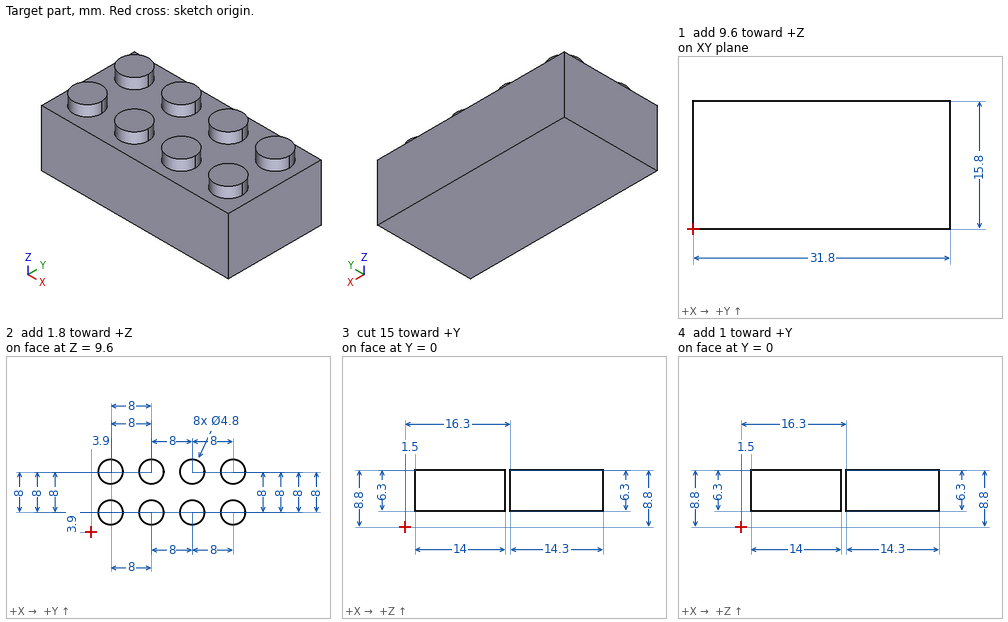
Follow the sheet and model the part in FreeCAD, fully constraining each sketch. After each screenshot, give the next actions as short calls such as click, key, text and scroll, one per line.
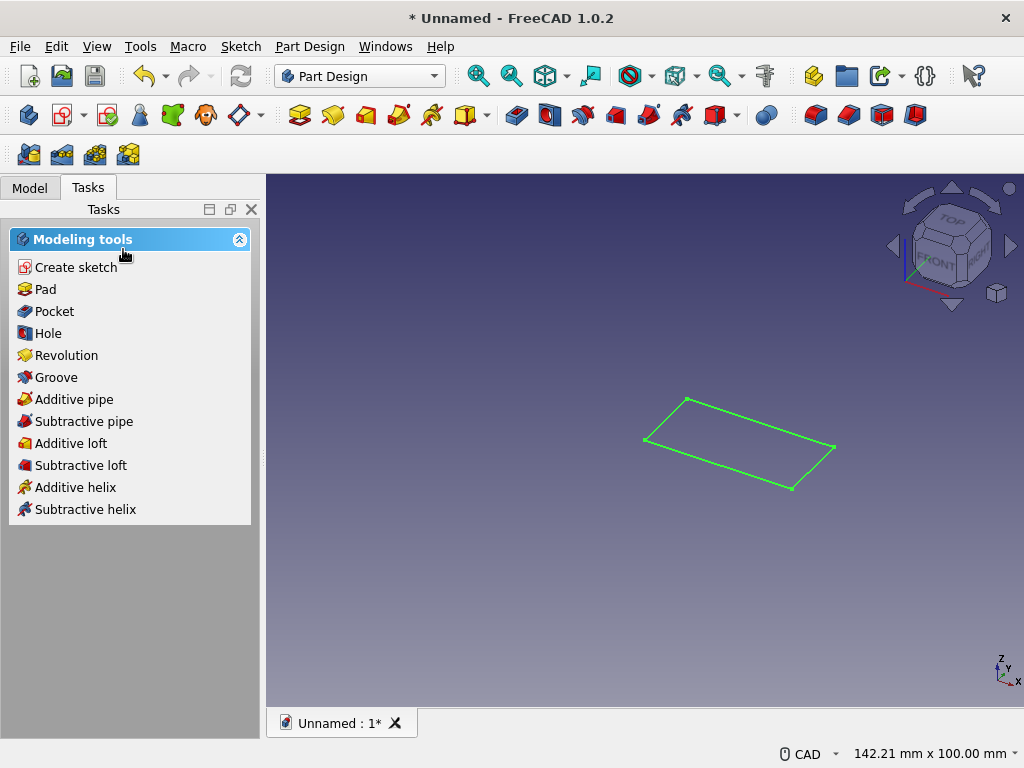
click(300, 116)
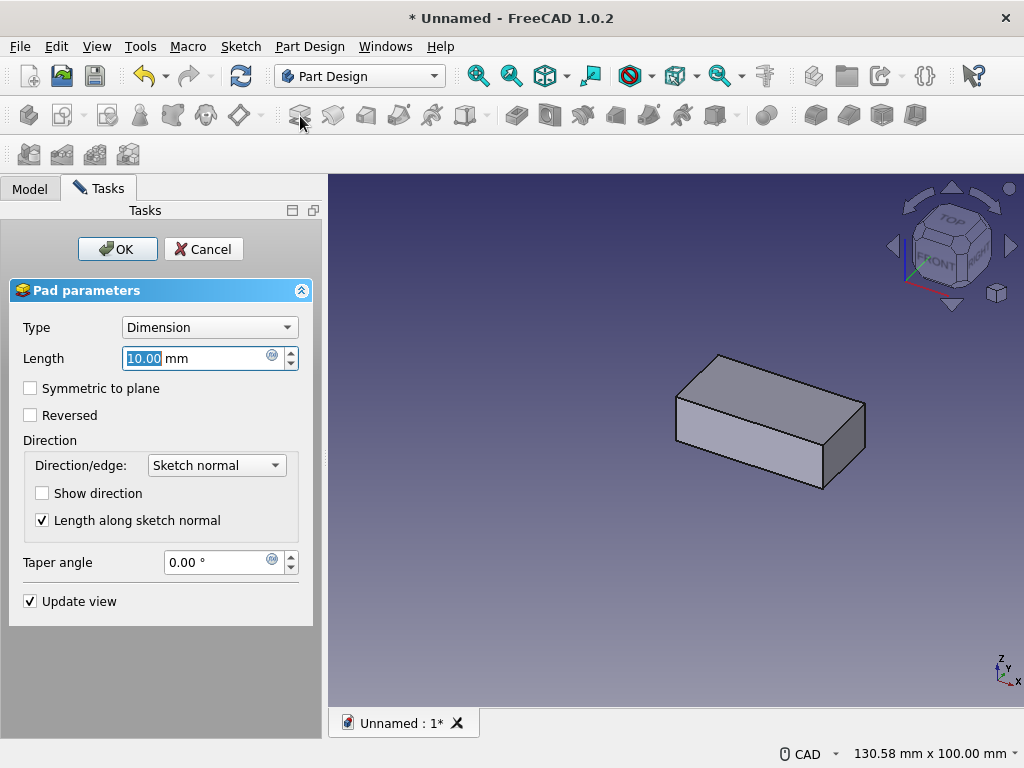
text(9.6)
key(Tab)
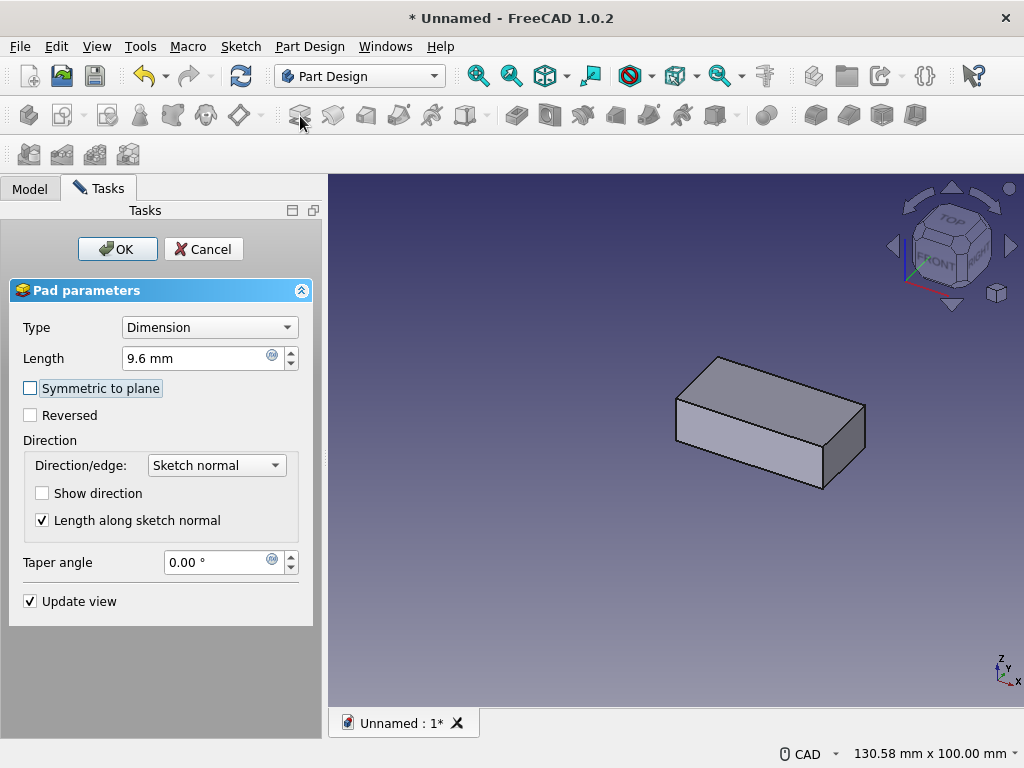
click(118, 249)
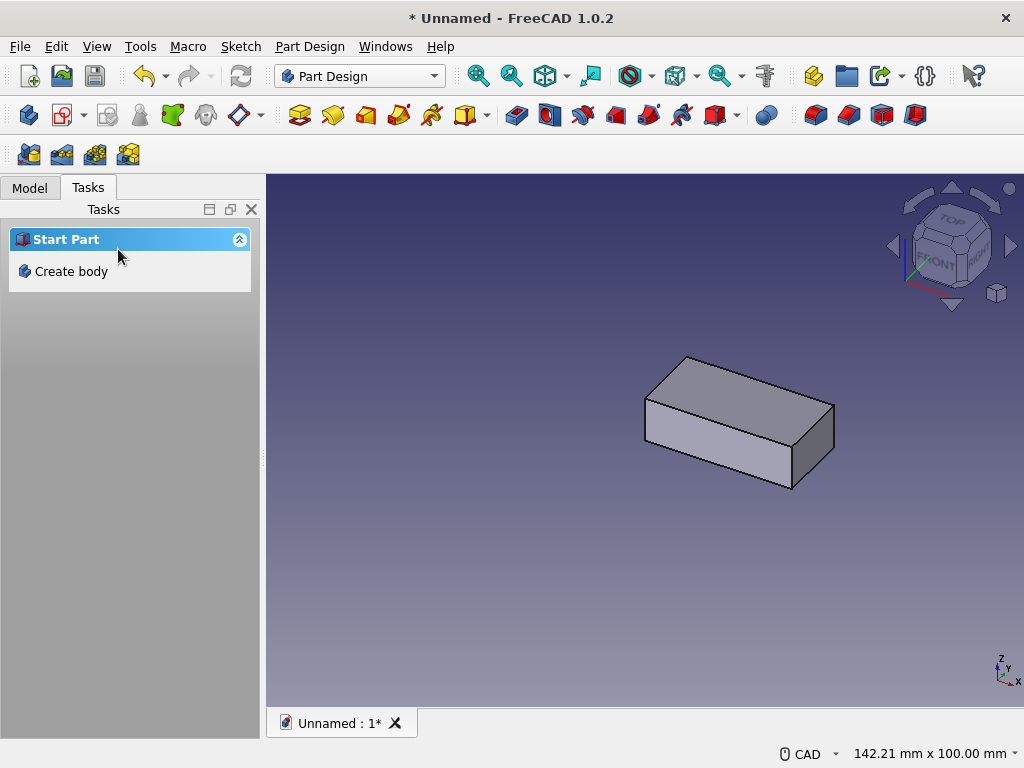
key(v)
key(f)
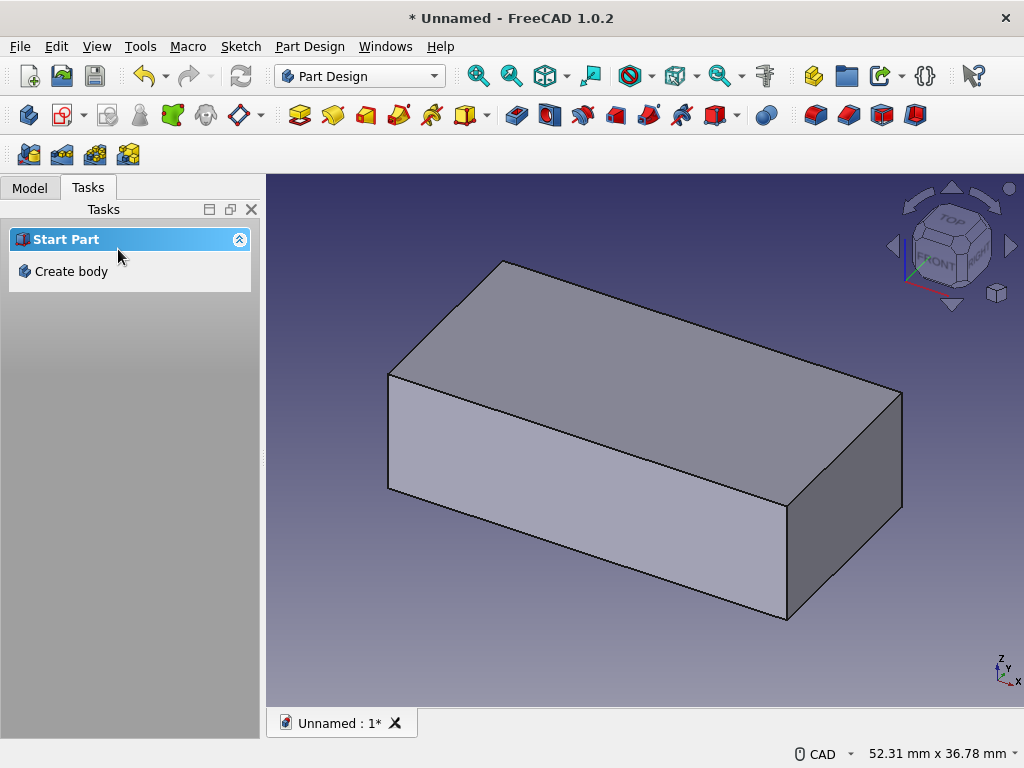
click(702, 401)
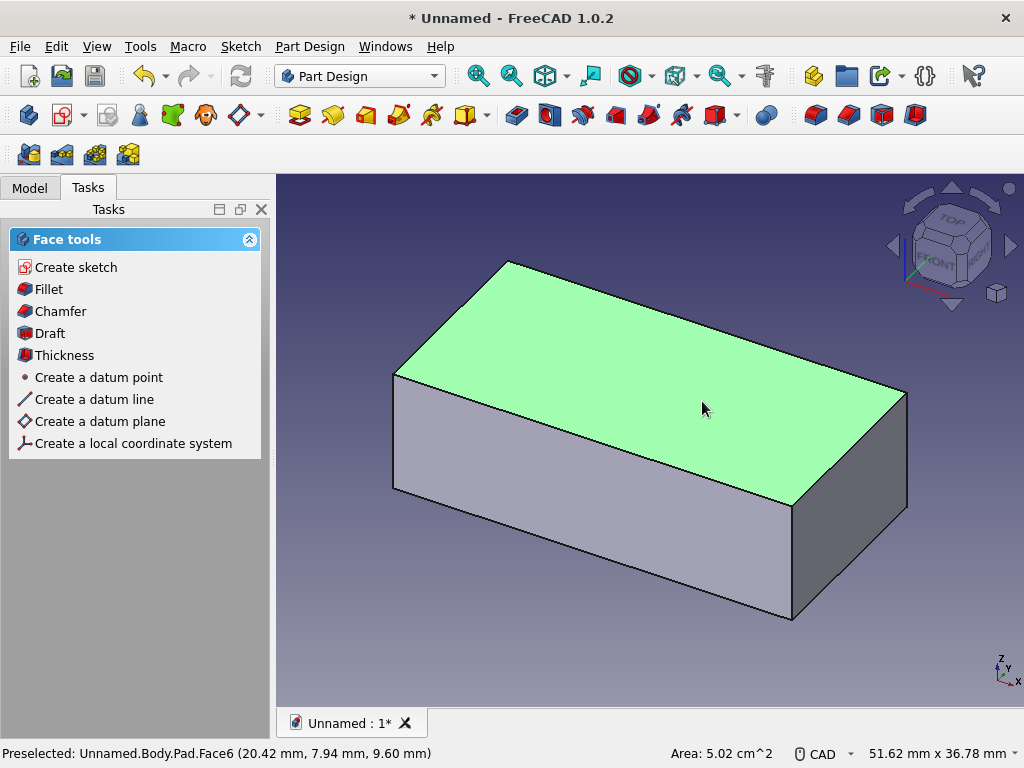
click(62, 116)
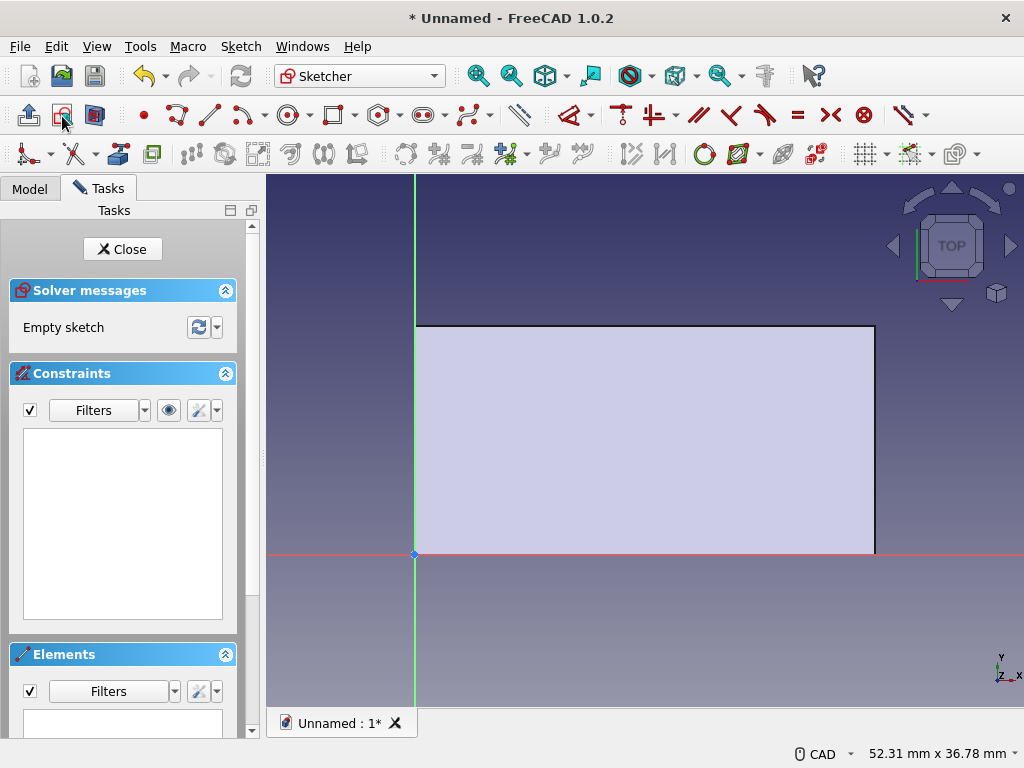
scroll(316, 391, down, 1)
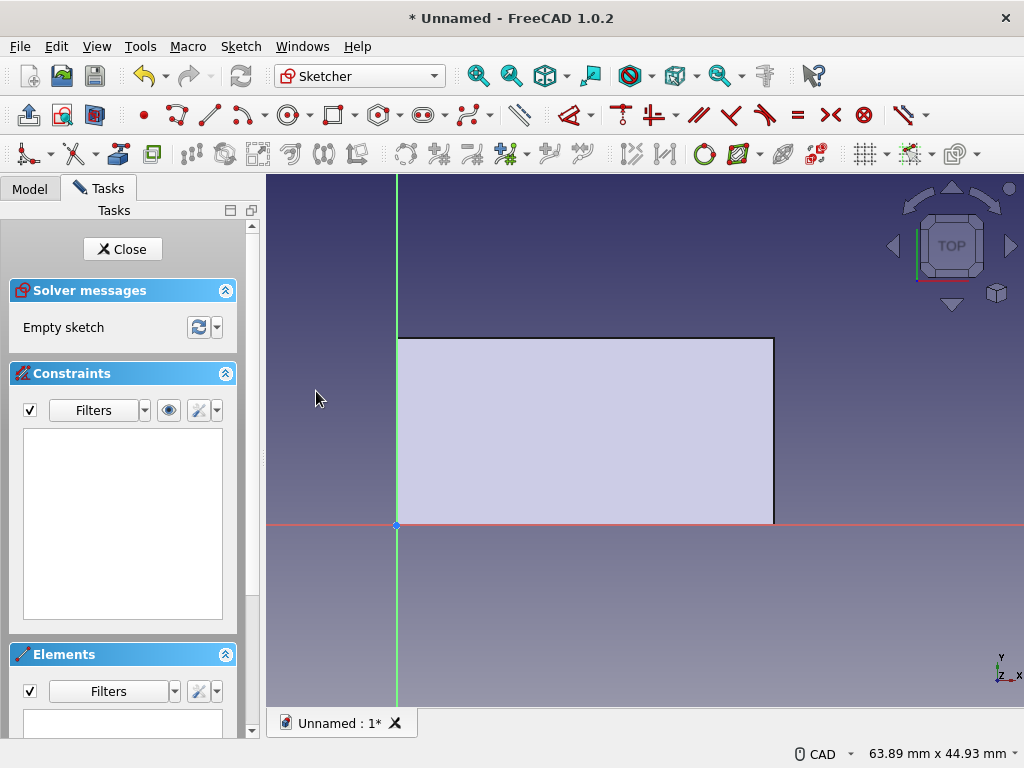
key(g)
key(c)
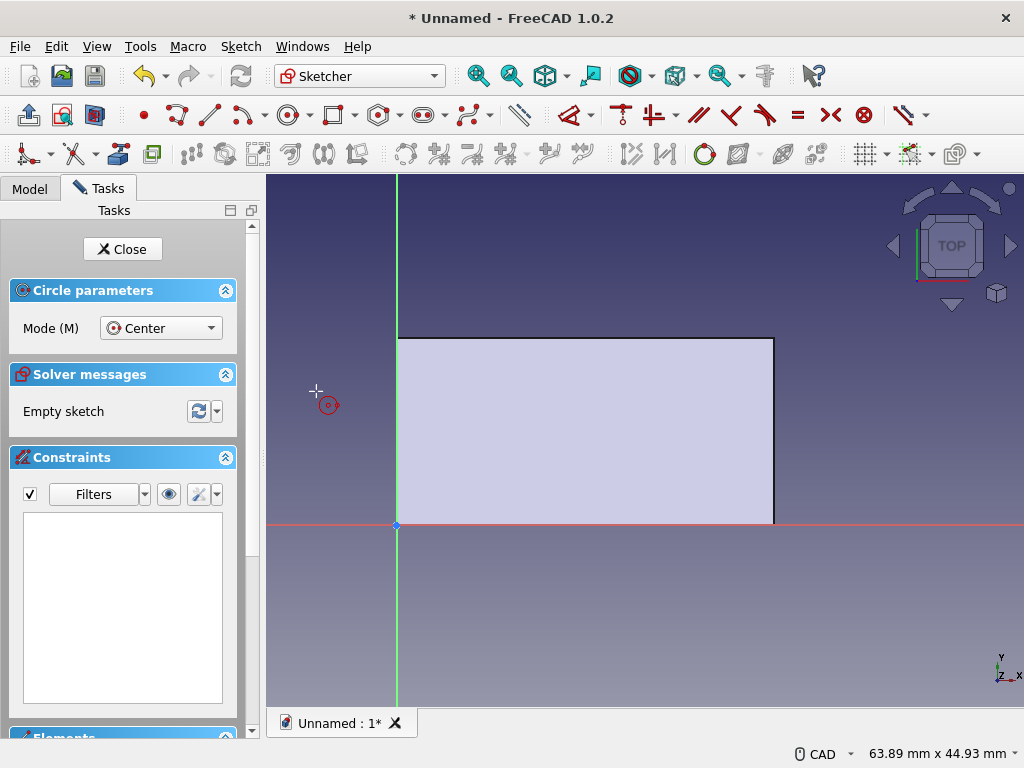
click(443, 384)
click(463, 364)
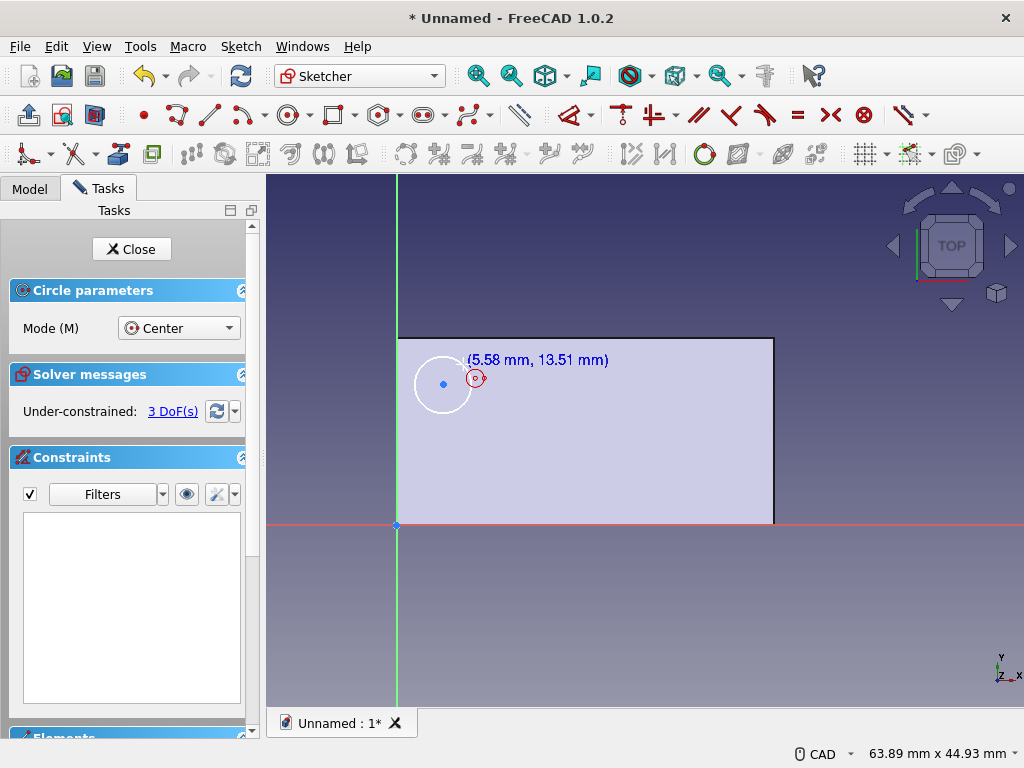
click(443, 479)
click(463, 459)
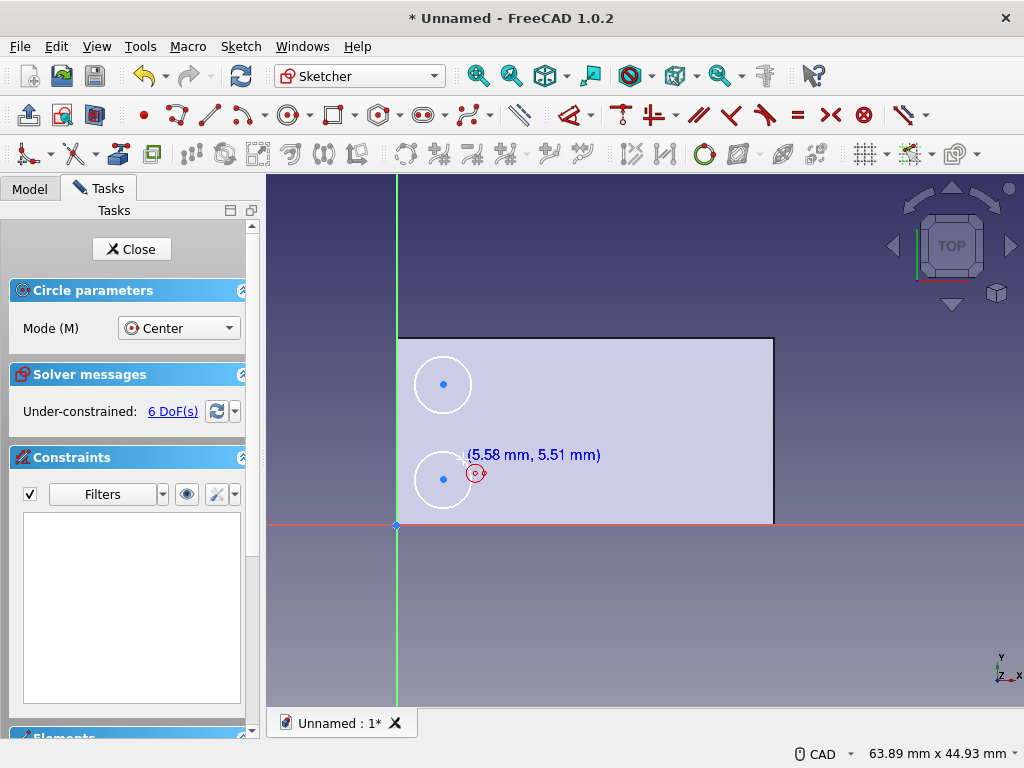
click(538, 384)
click(558, 364)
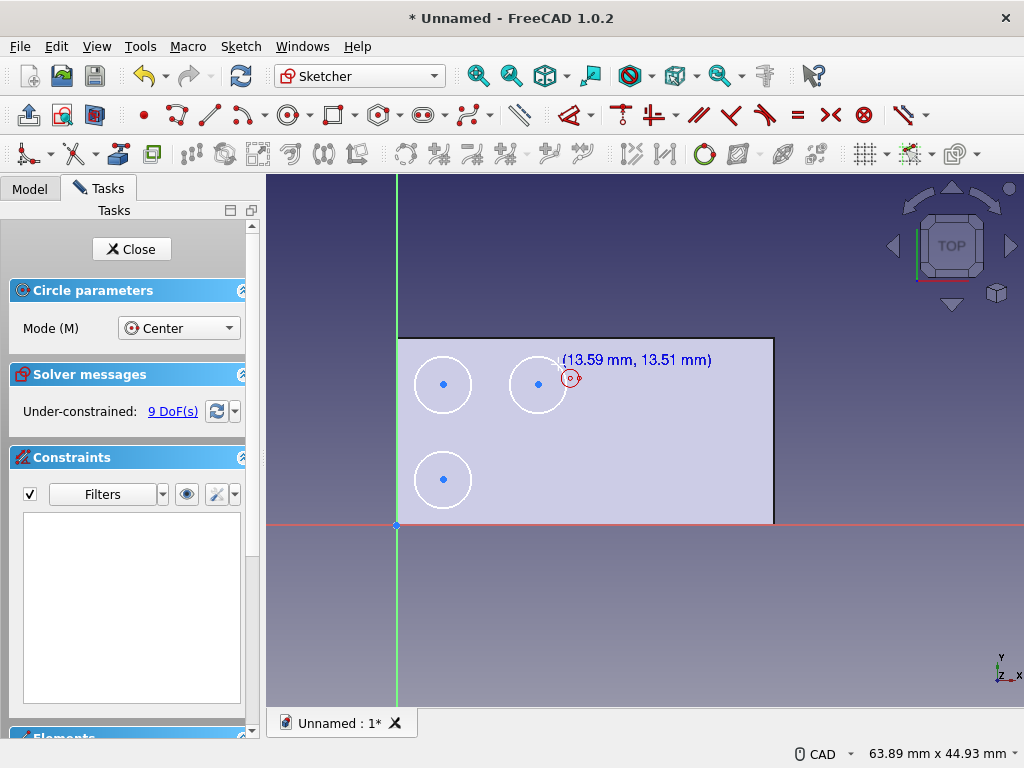
click(633, 384)
click(653, 364)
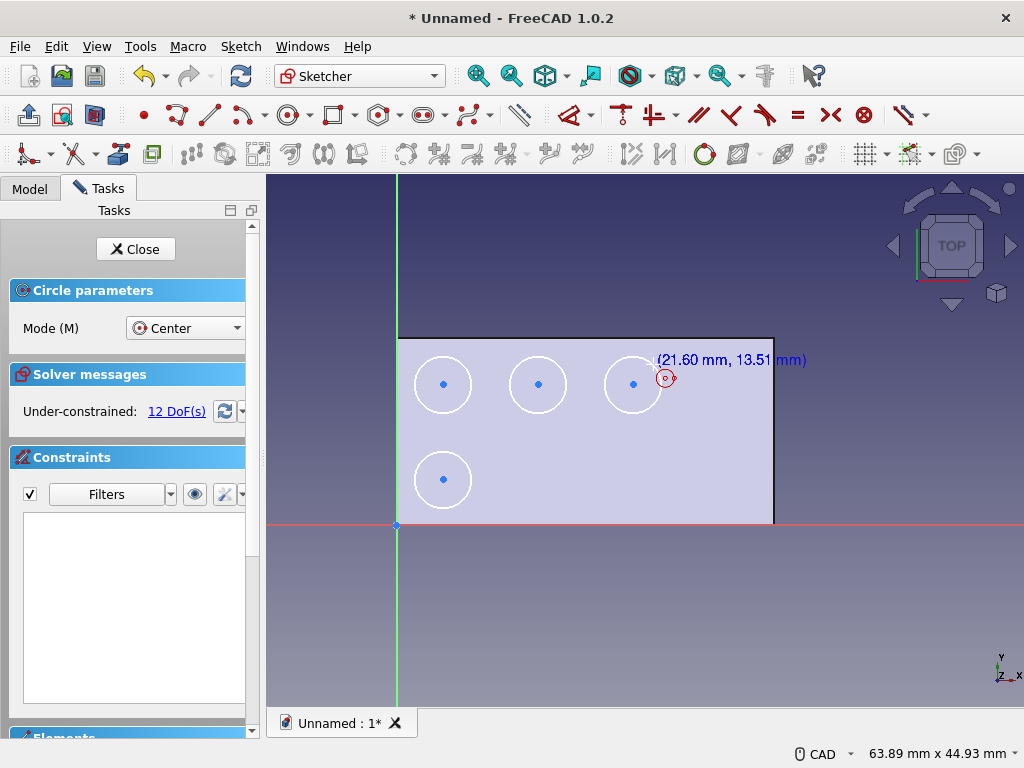
click(728, 384)
click(748, 364)